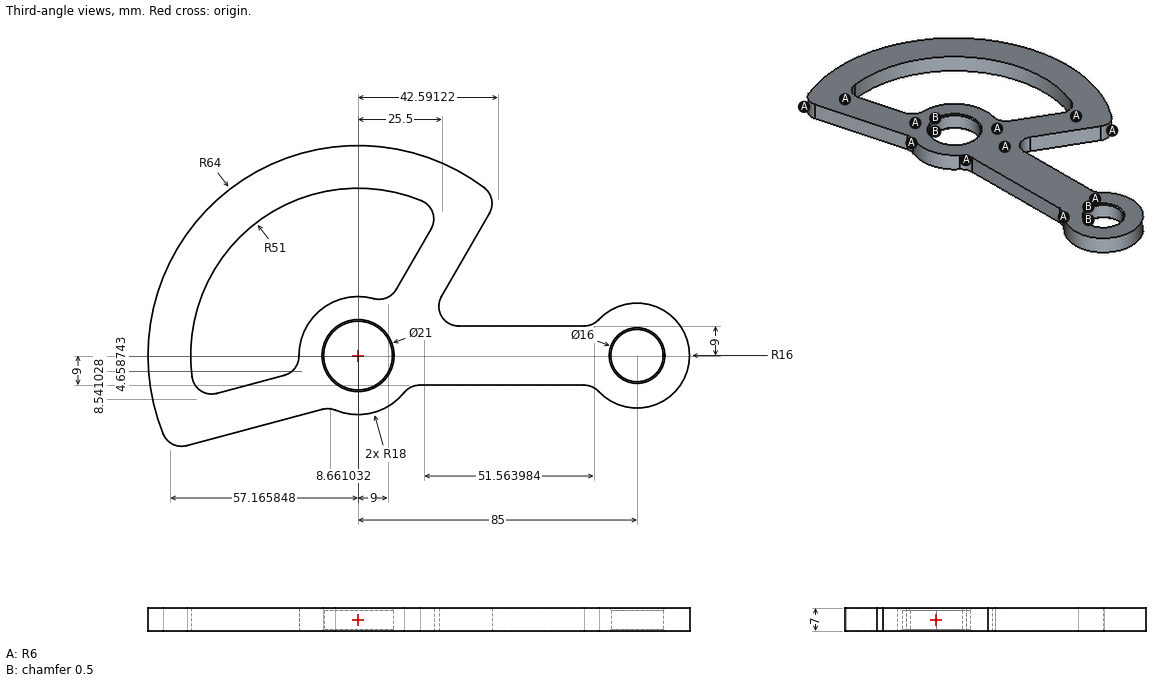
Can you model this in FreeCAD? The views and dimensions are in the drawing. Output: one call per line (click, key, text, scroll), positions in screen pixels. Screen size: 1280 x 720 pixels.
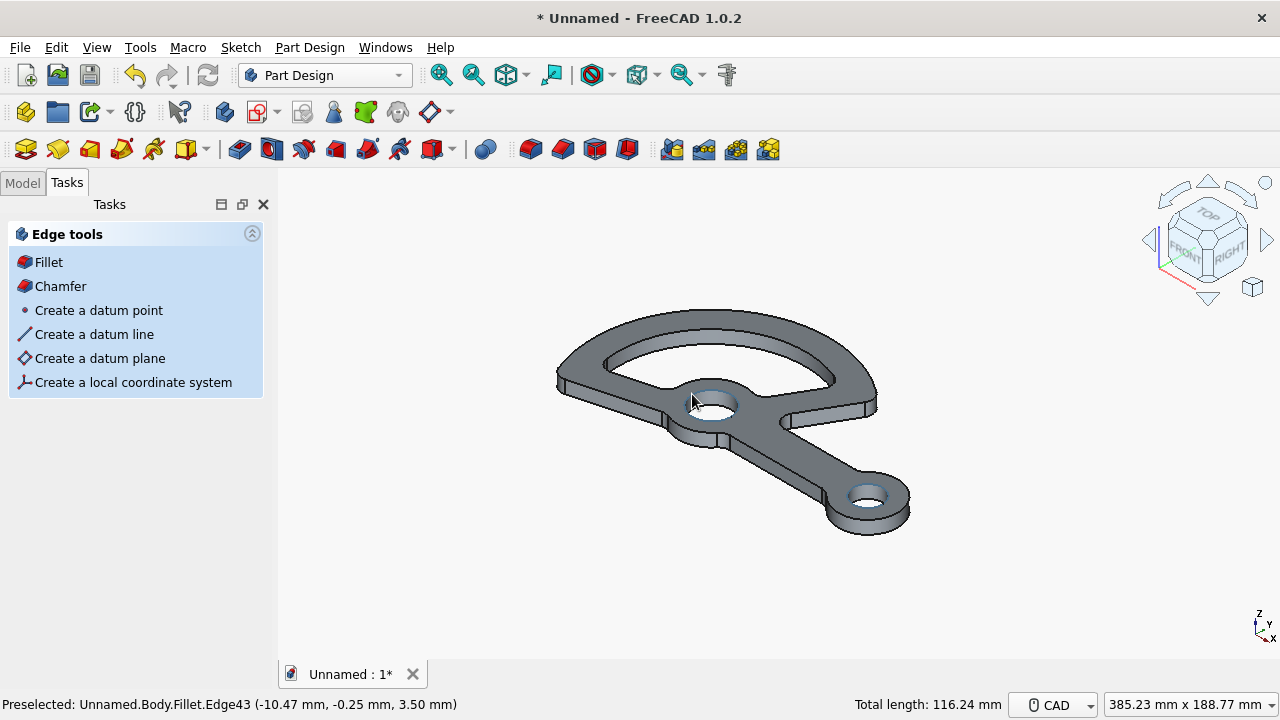
key(2)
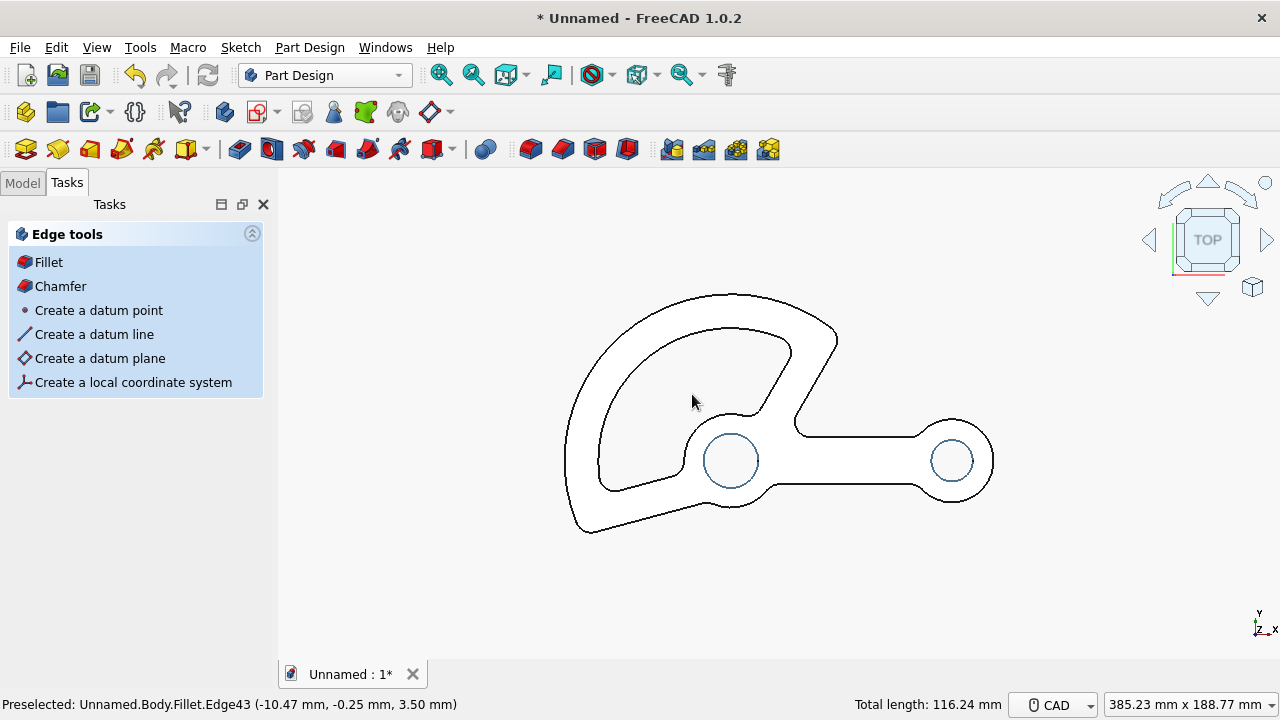
key(0)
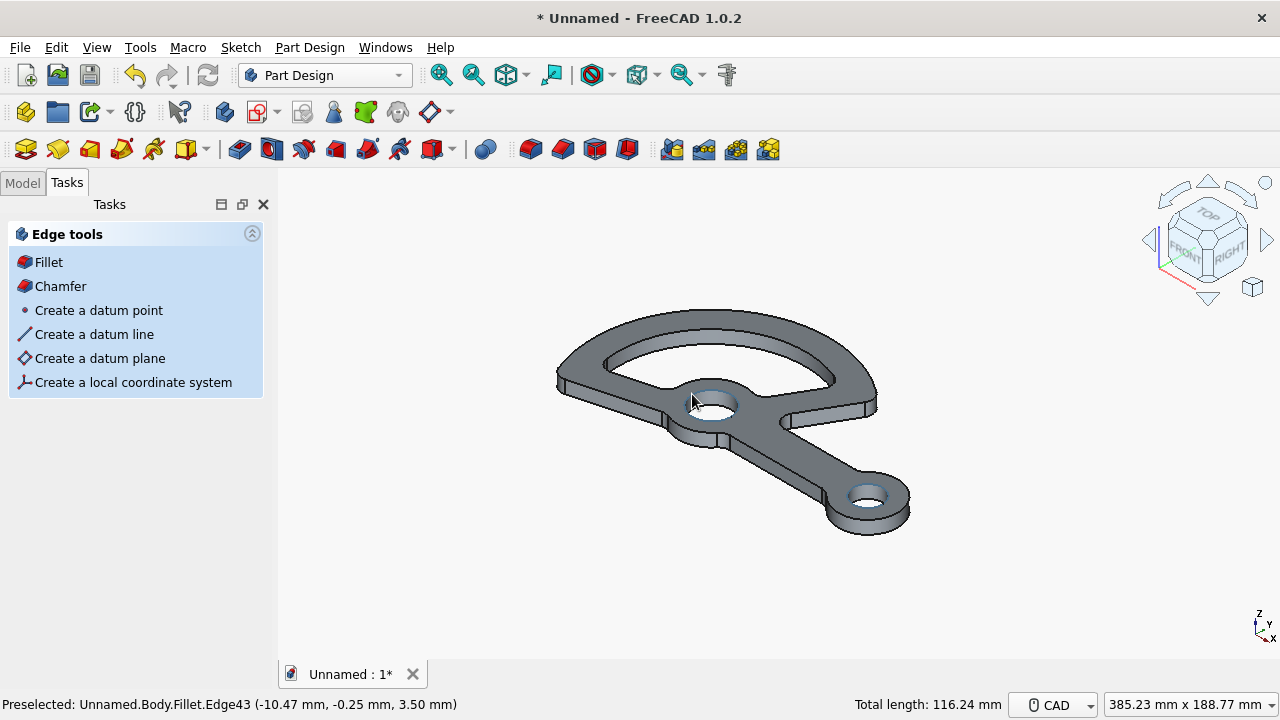
key(1)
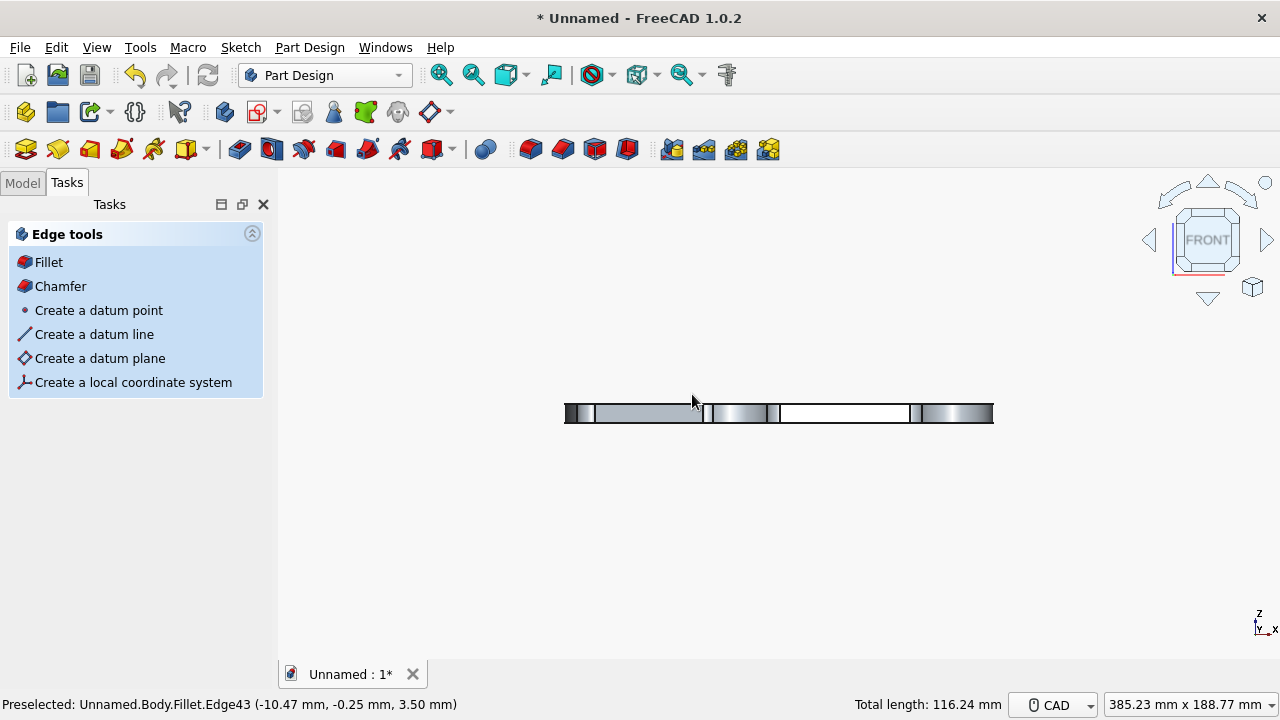
click(442, 76)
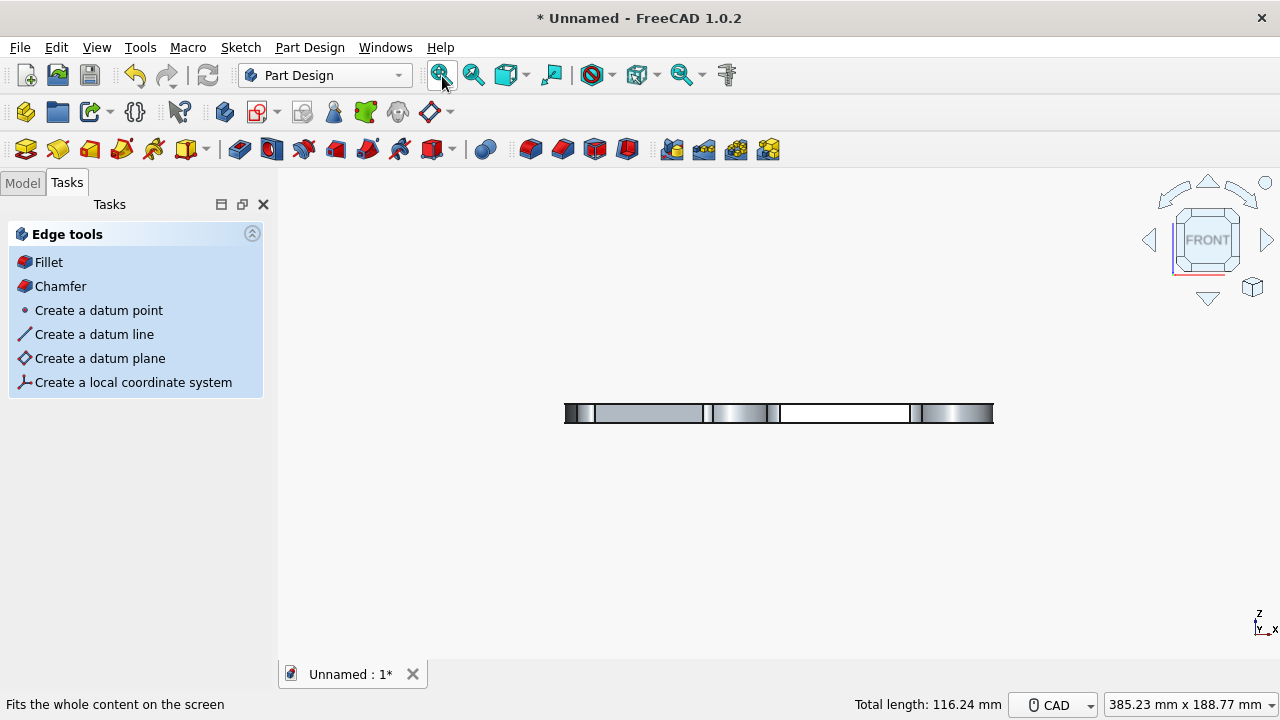
key(3)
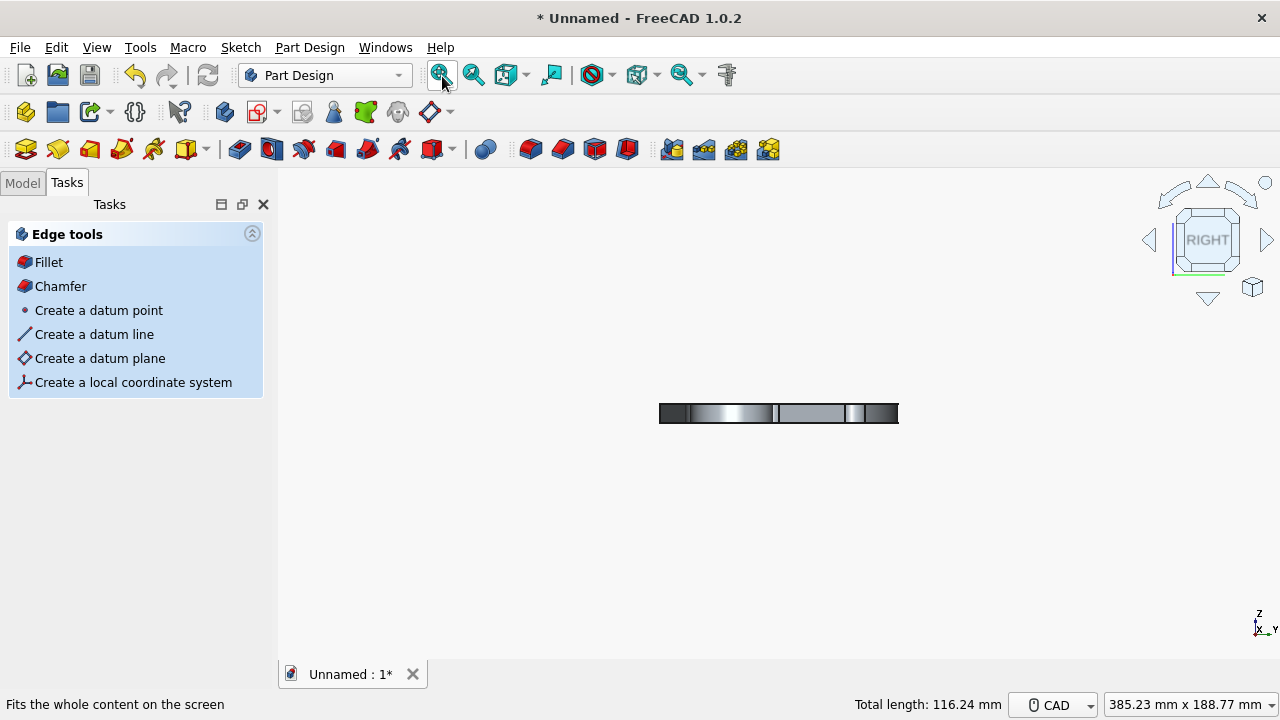
click(442, 76)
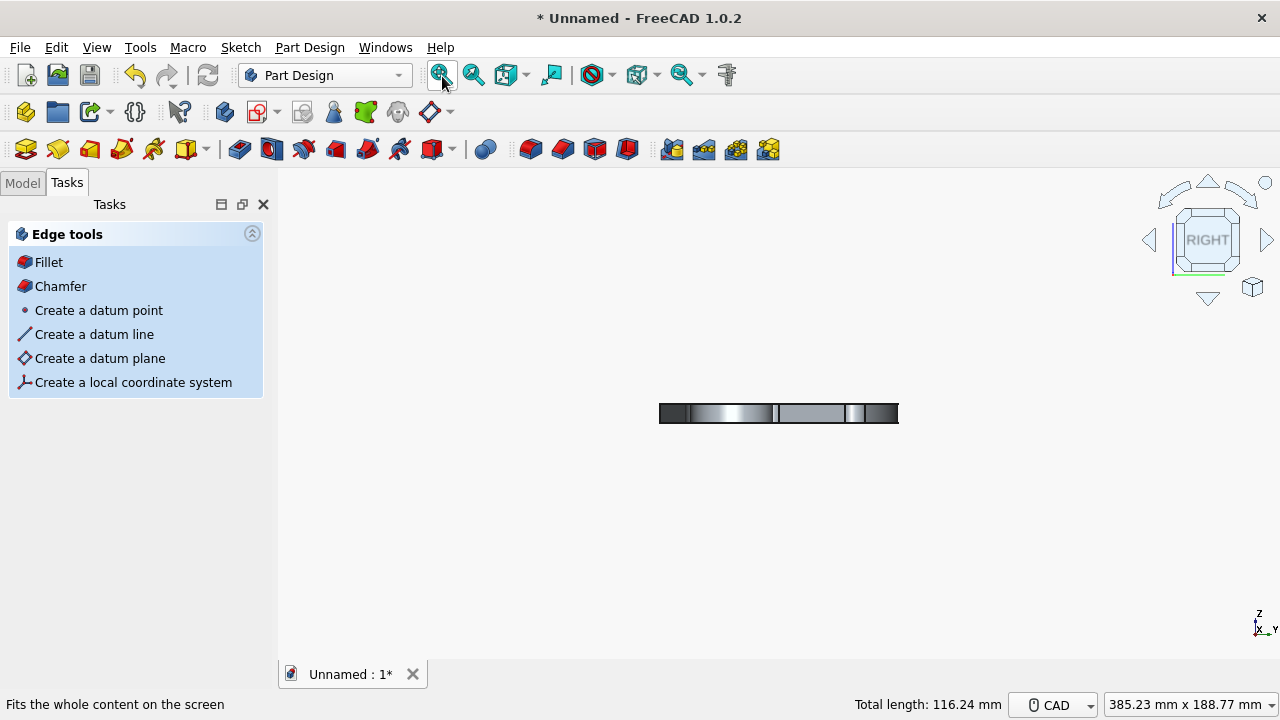
key(5)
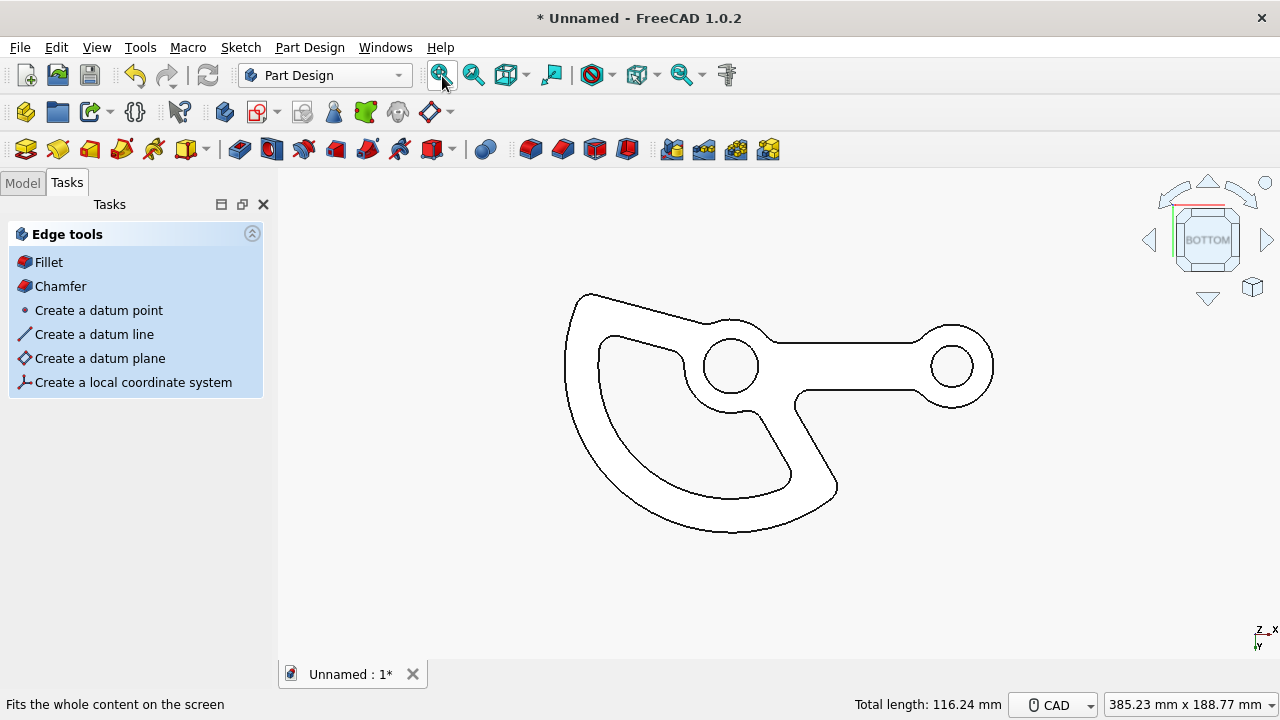
click(931, 365, ctrl)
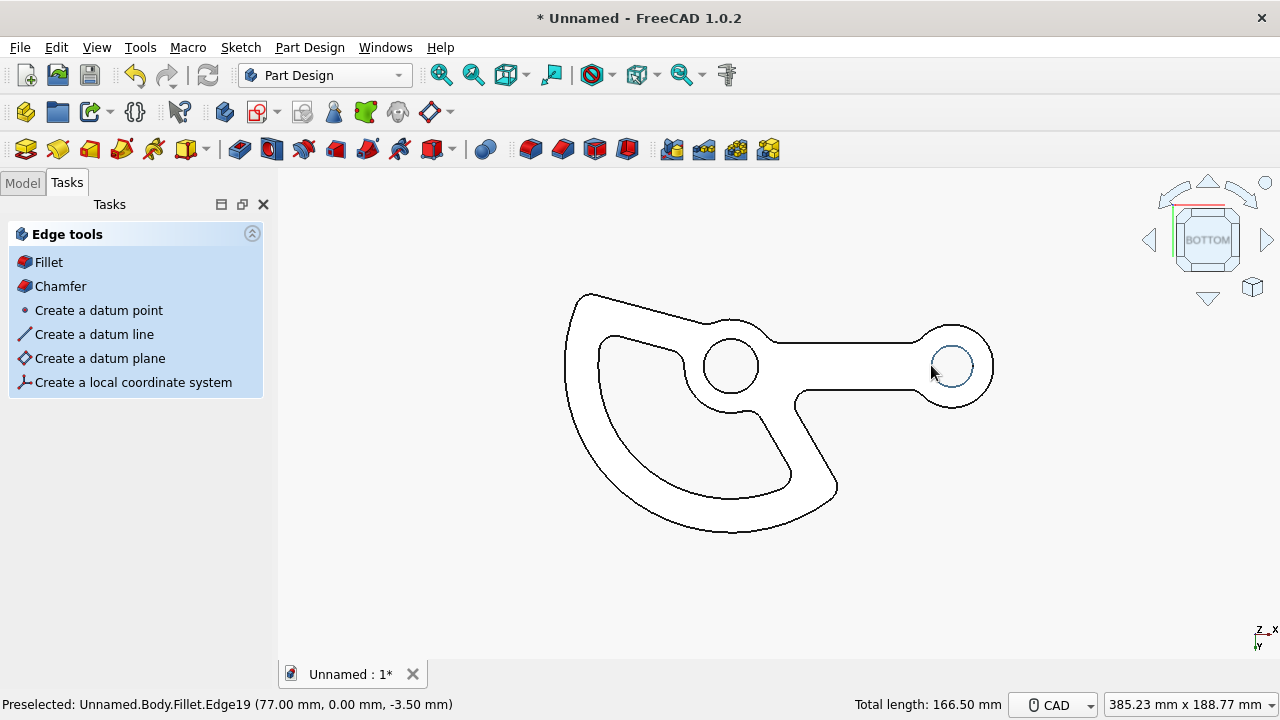
click(704, 365, ctrl)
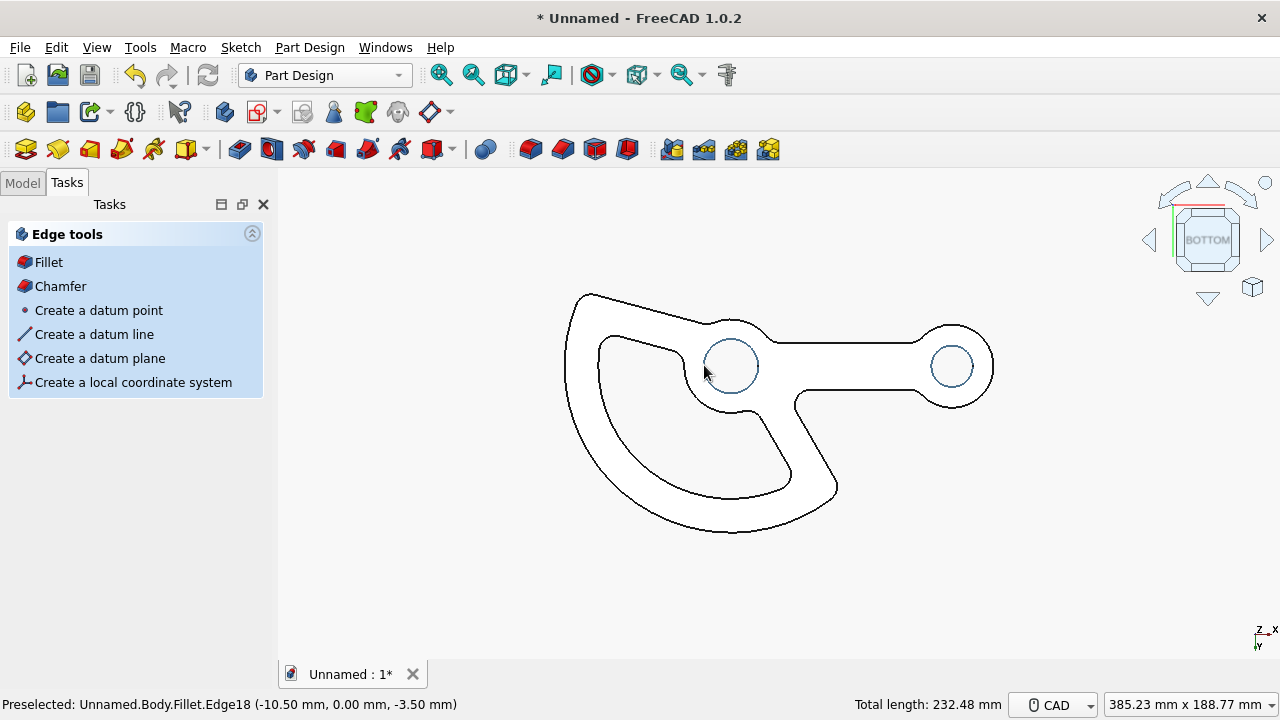
click(564, 150)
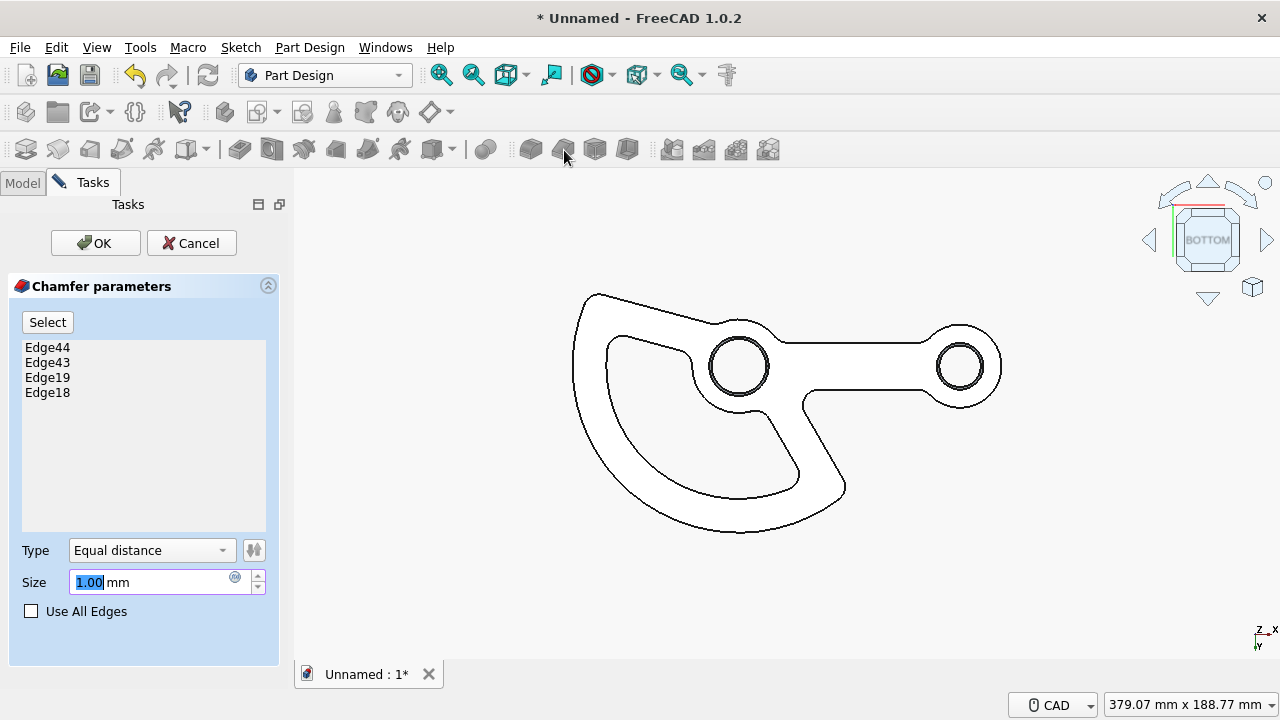
text(0.5)
key(Tab)